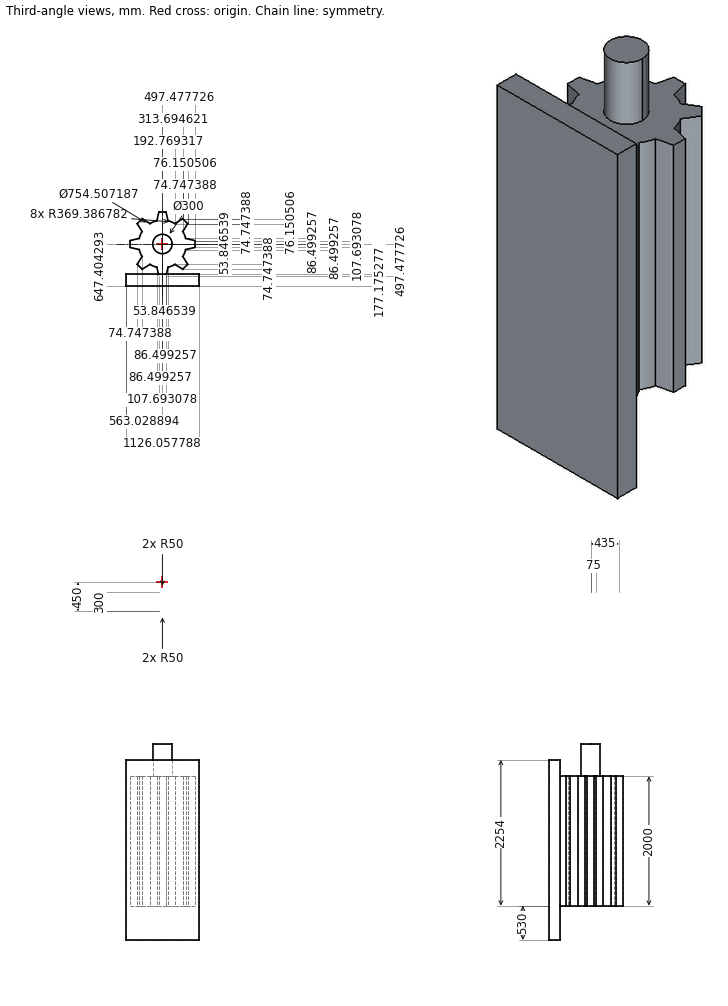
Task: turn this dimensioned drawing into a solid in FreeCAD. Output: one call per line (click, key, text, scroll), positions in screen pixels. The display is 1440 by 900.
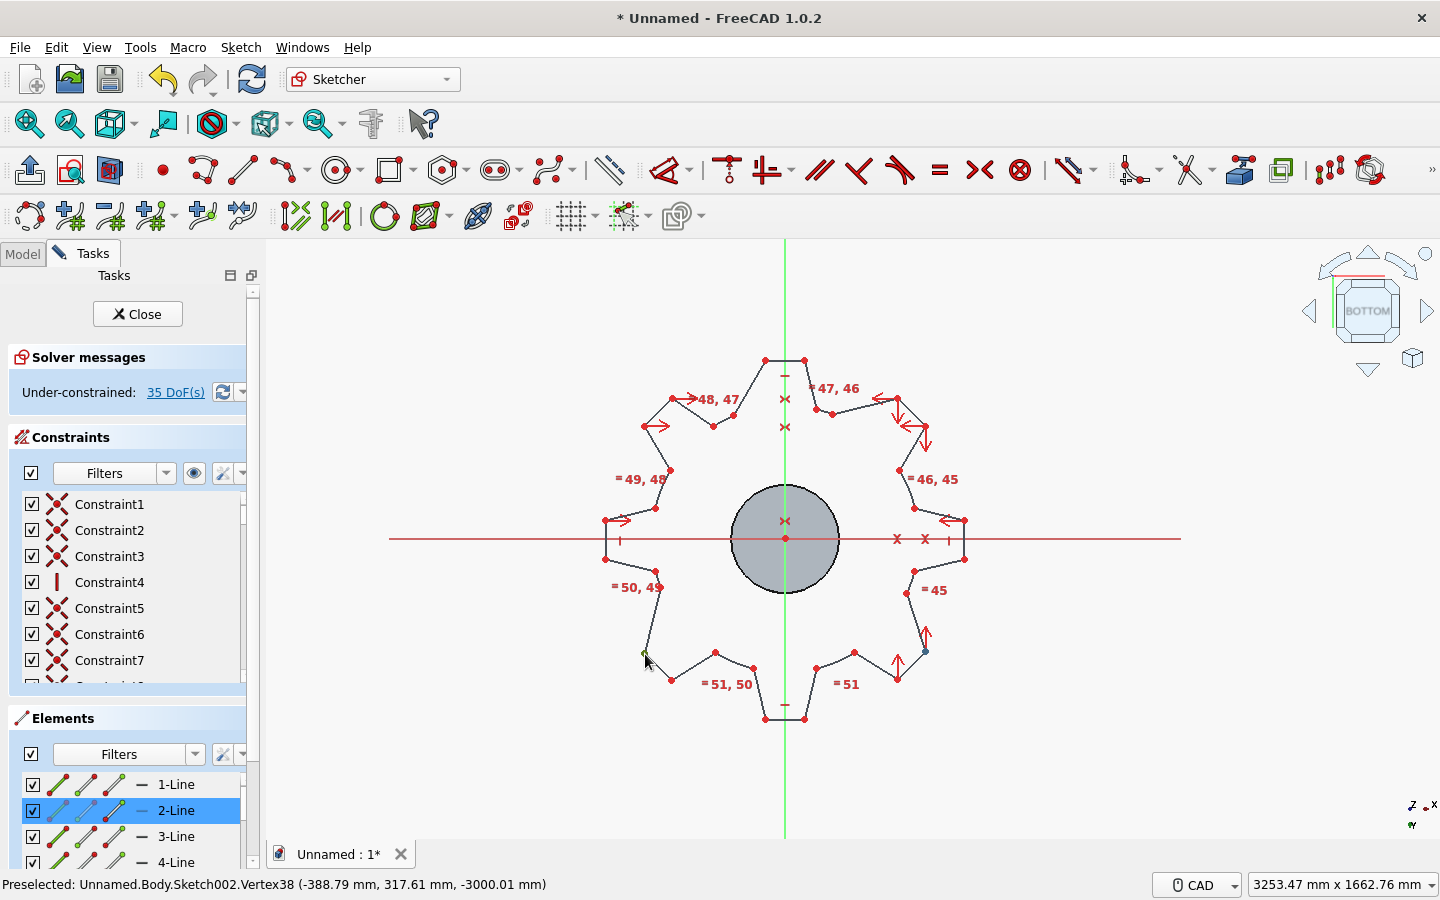
click(785, 772)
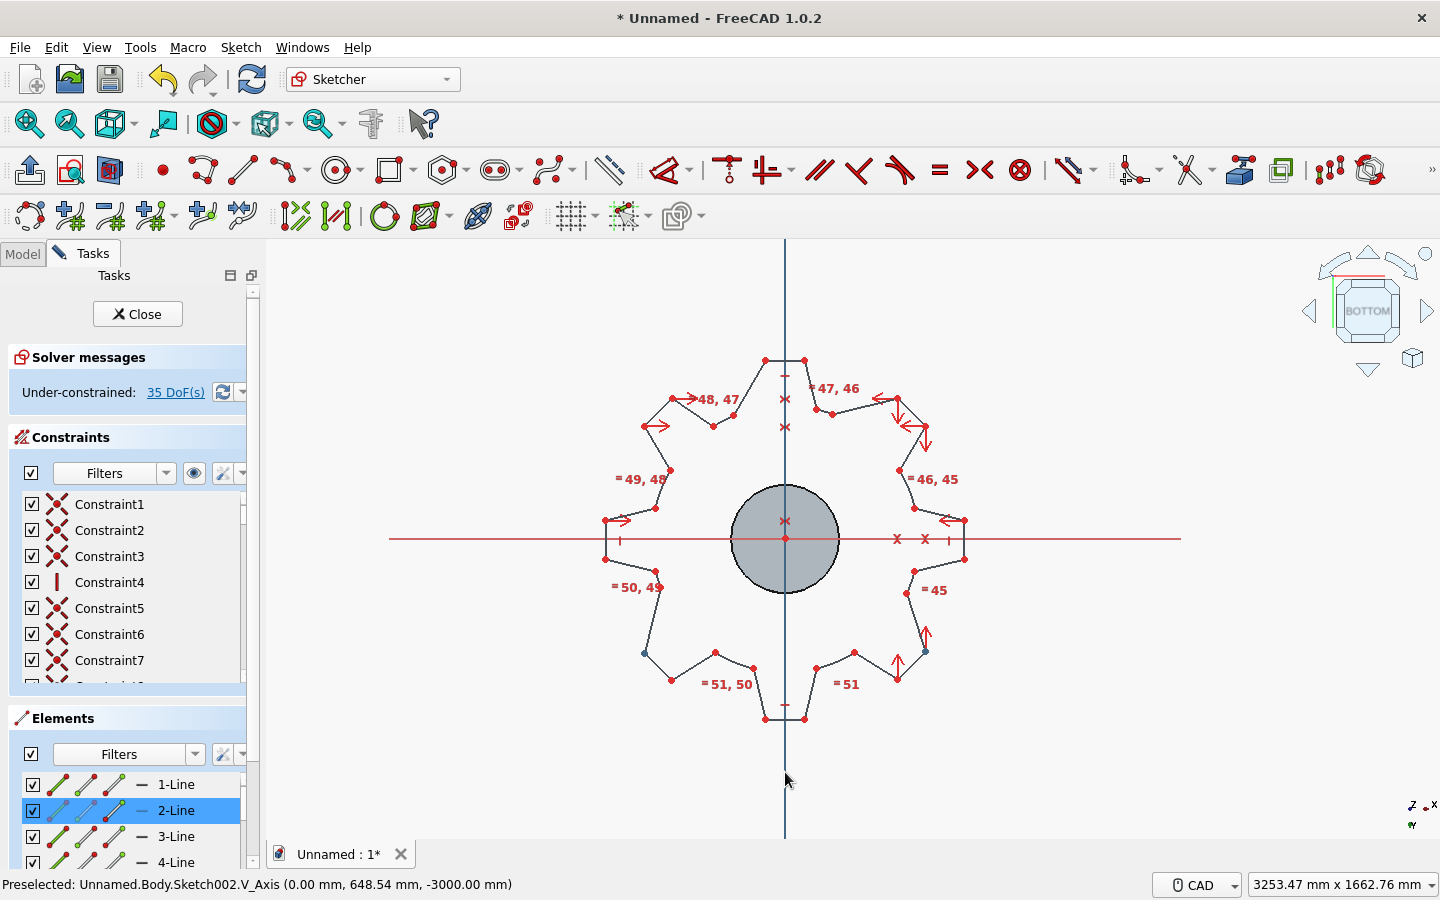
click(980, 170)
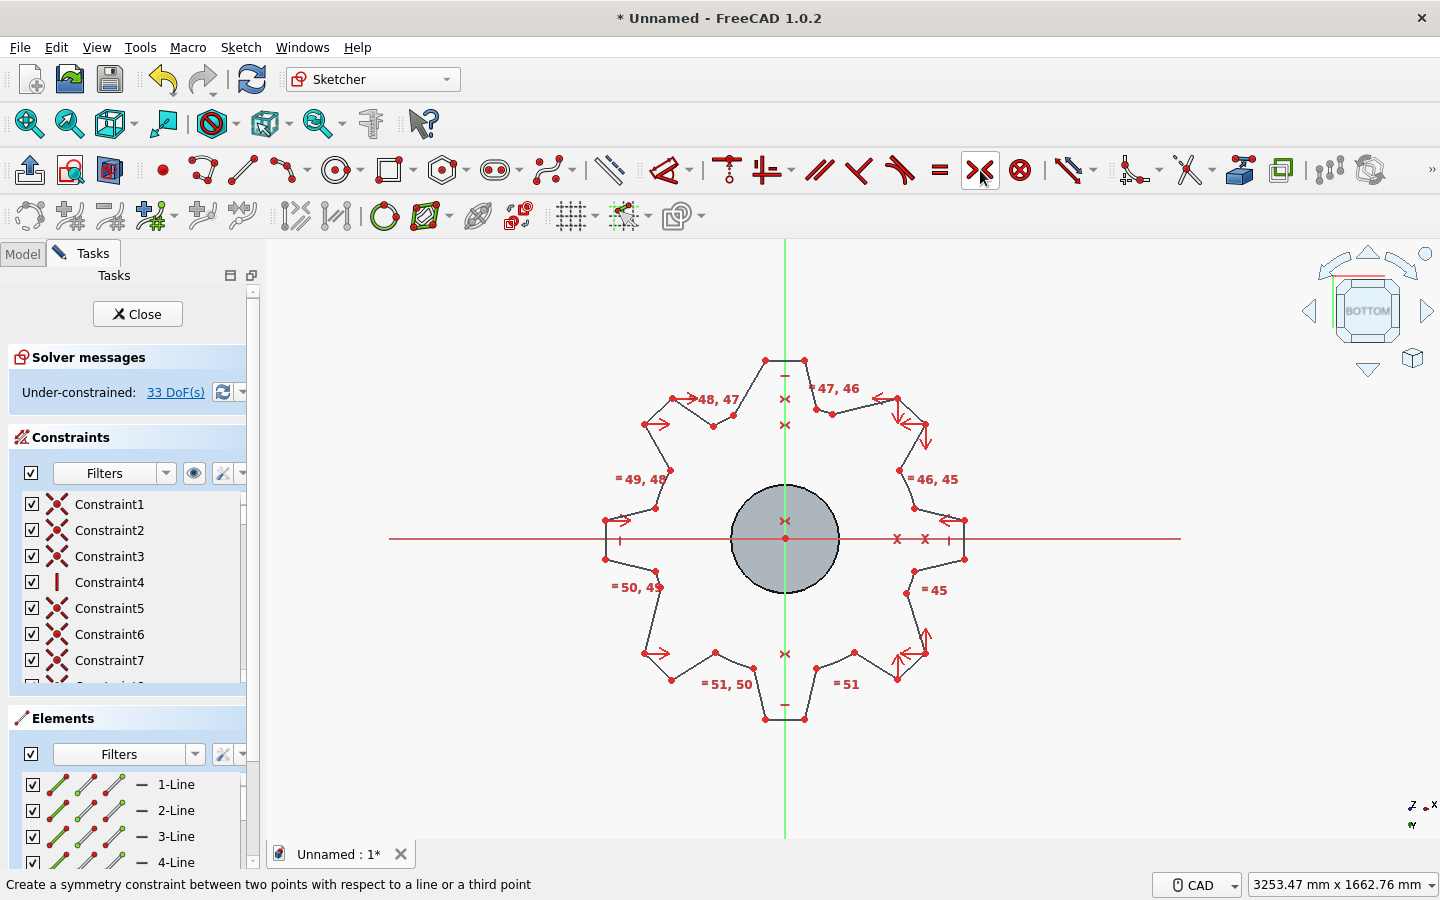
click(898, 679)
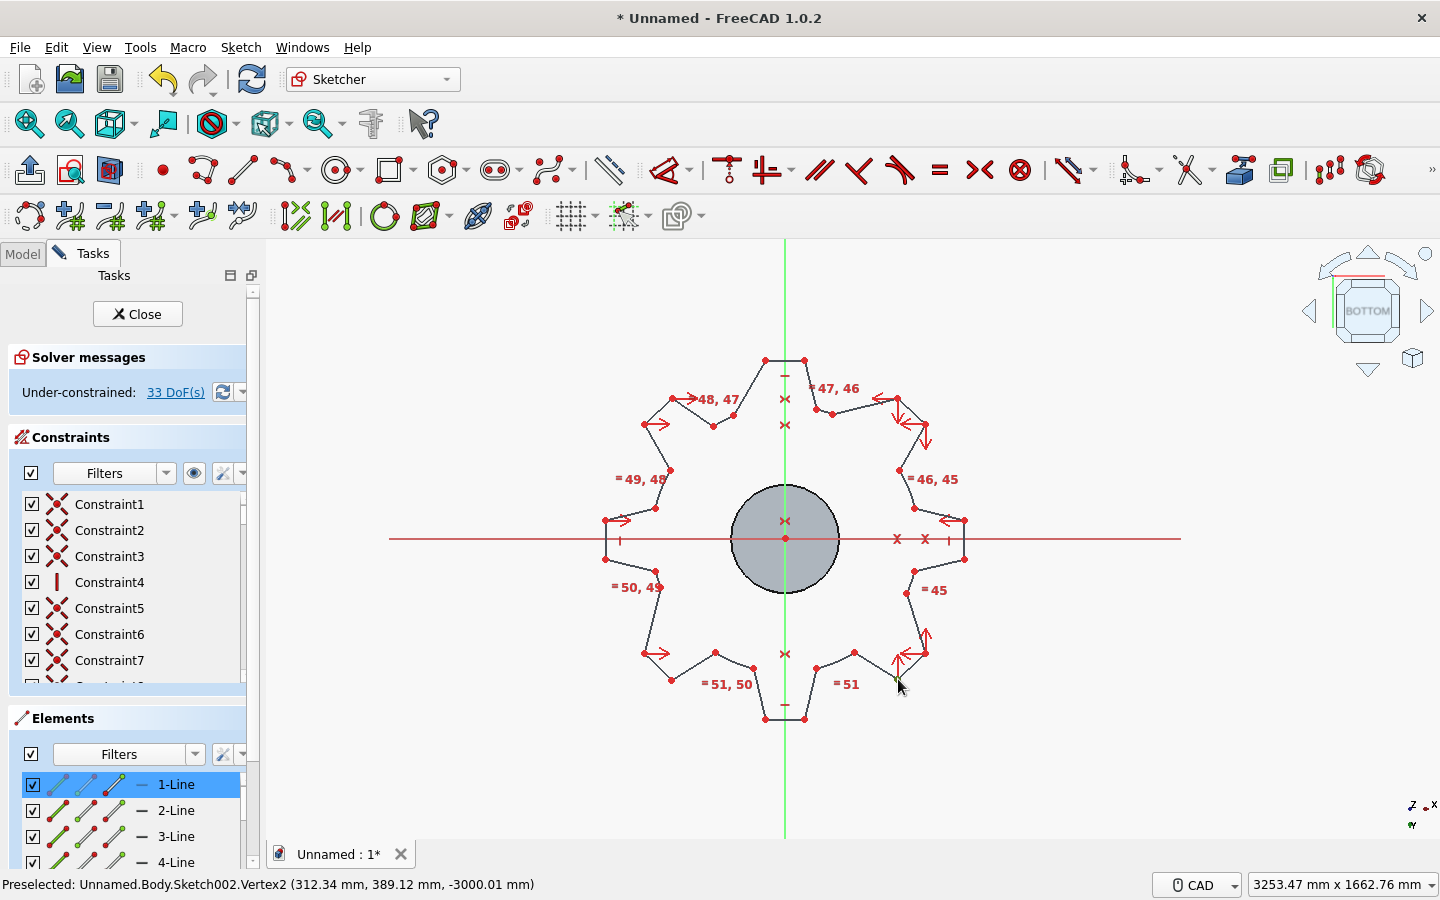
click(672, 681)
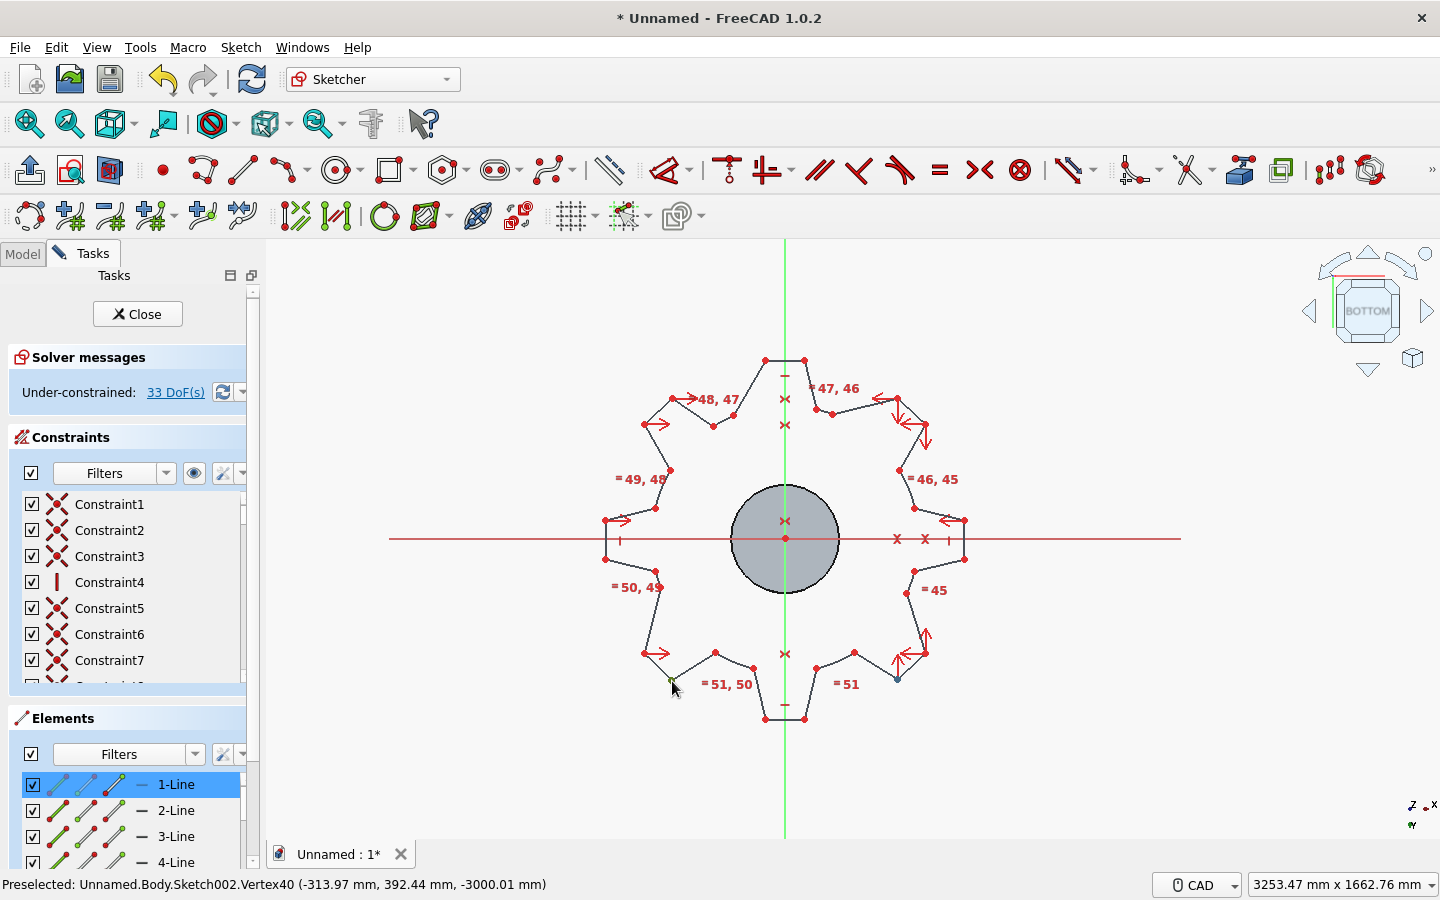
click(785, 772)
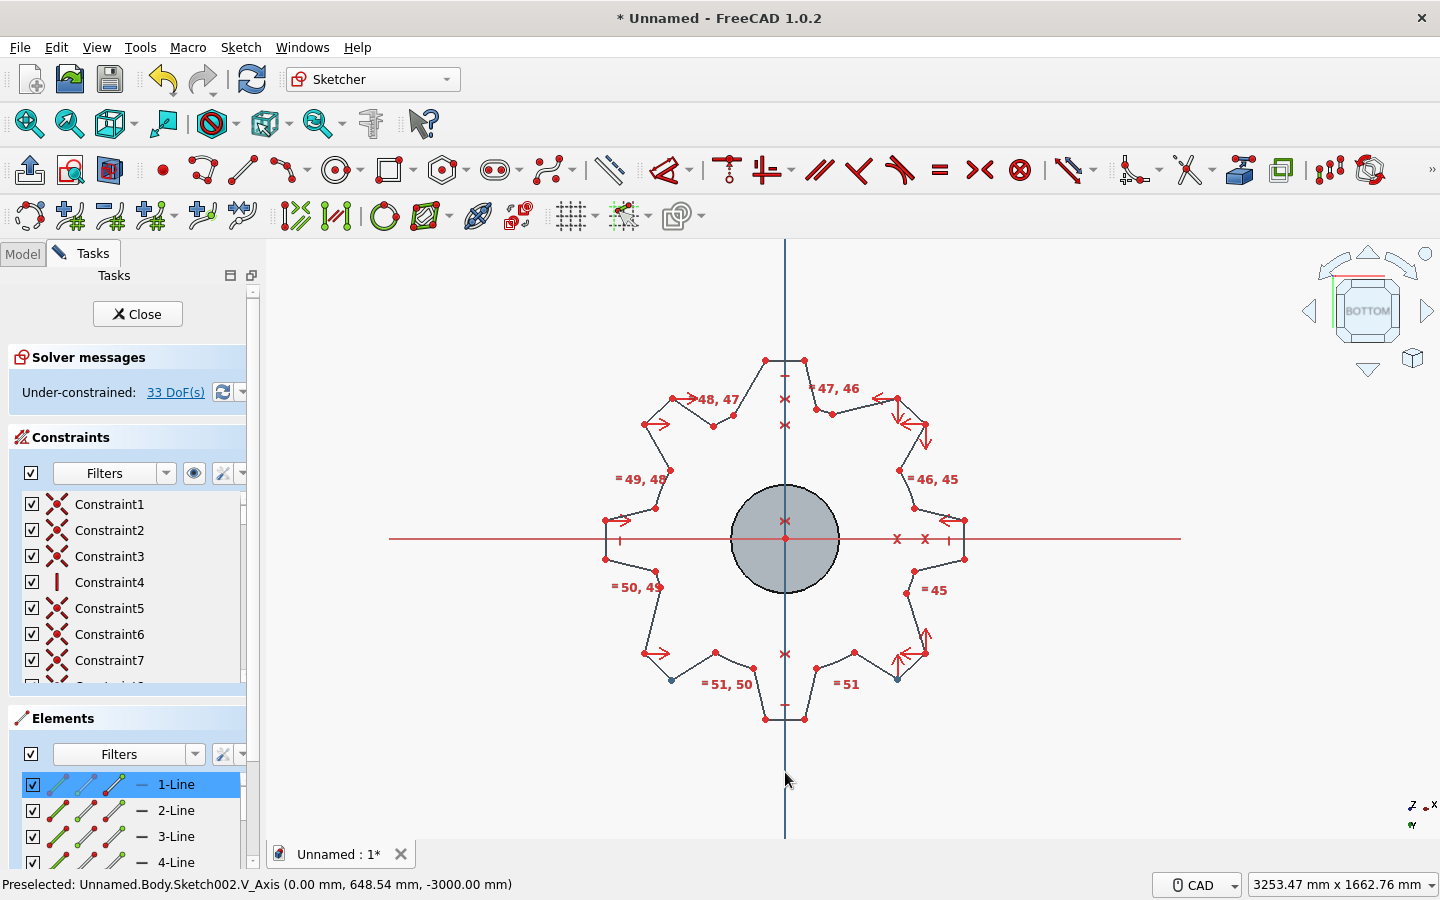
click(980, 170)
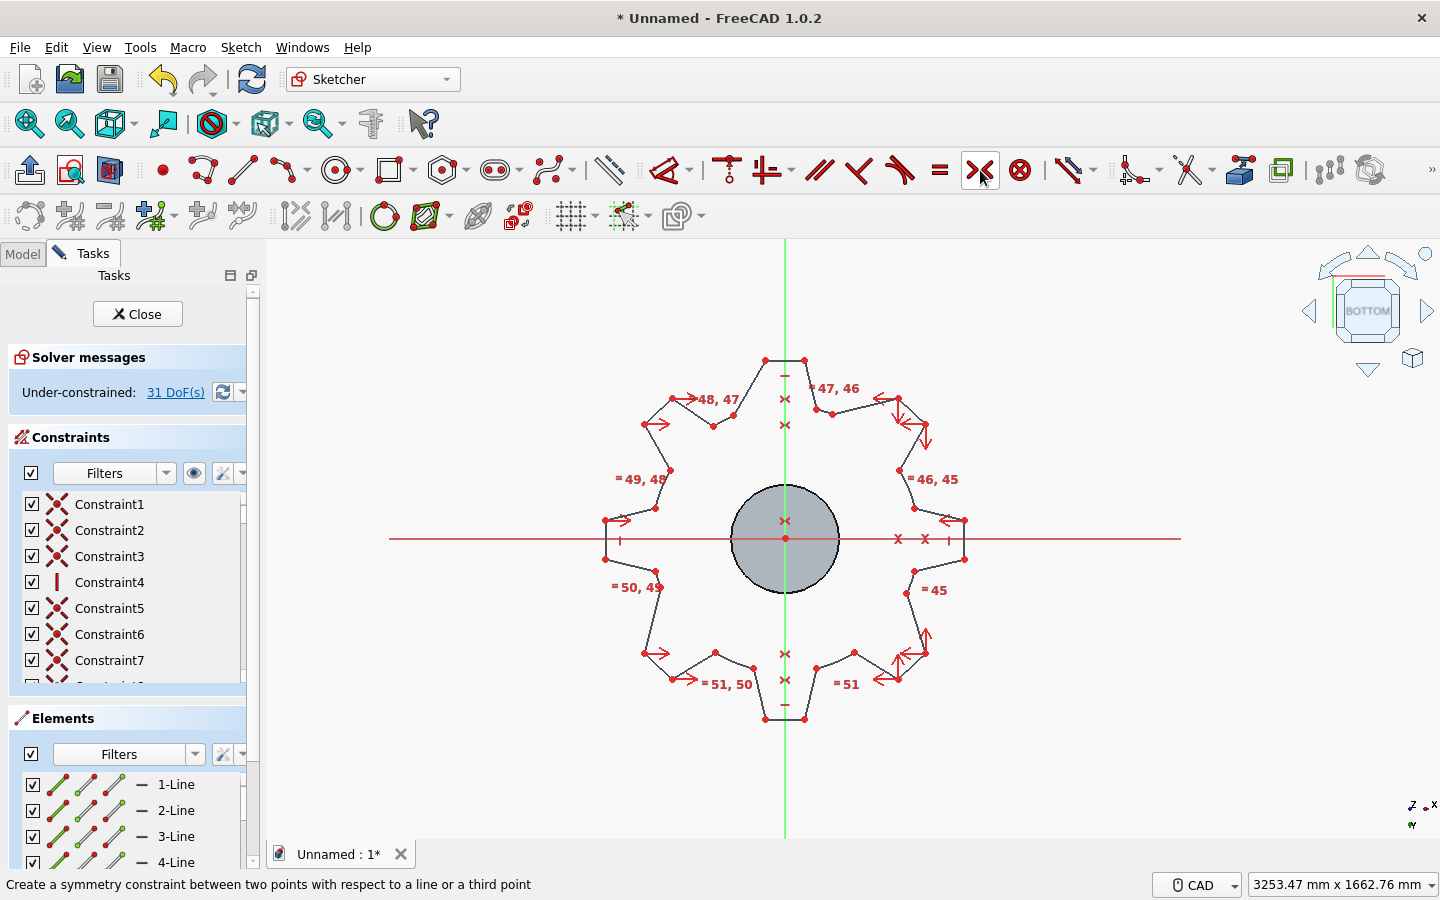
click(766, 361)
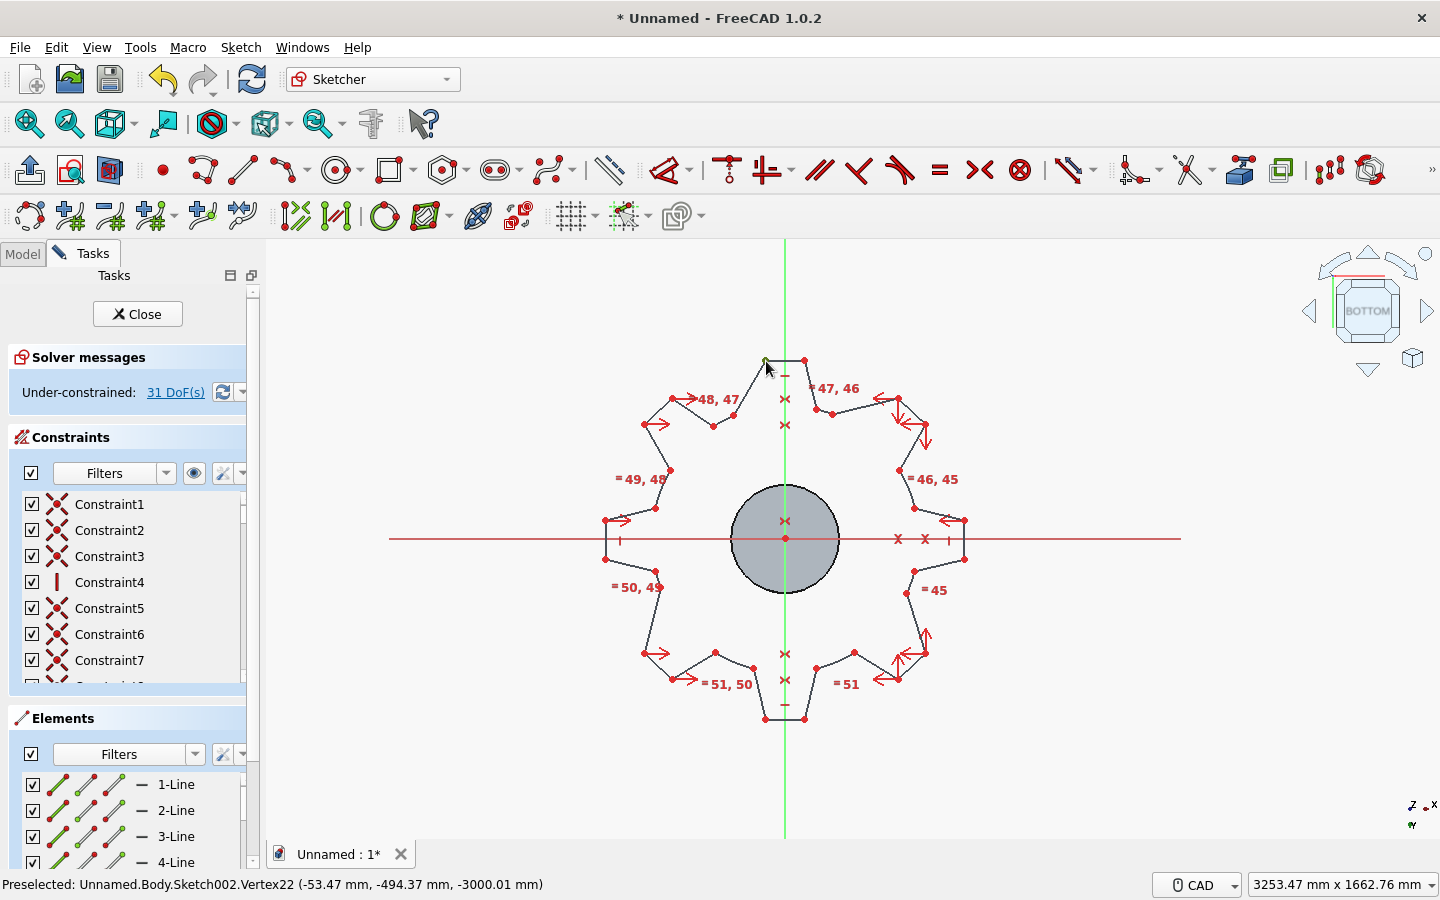
click(766, 720)